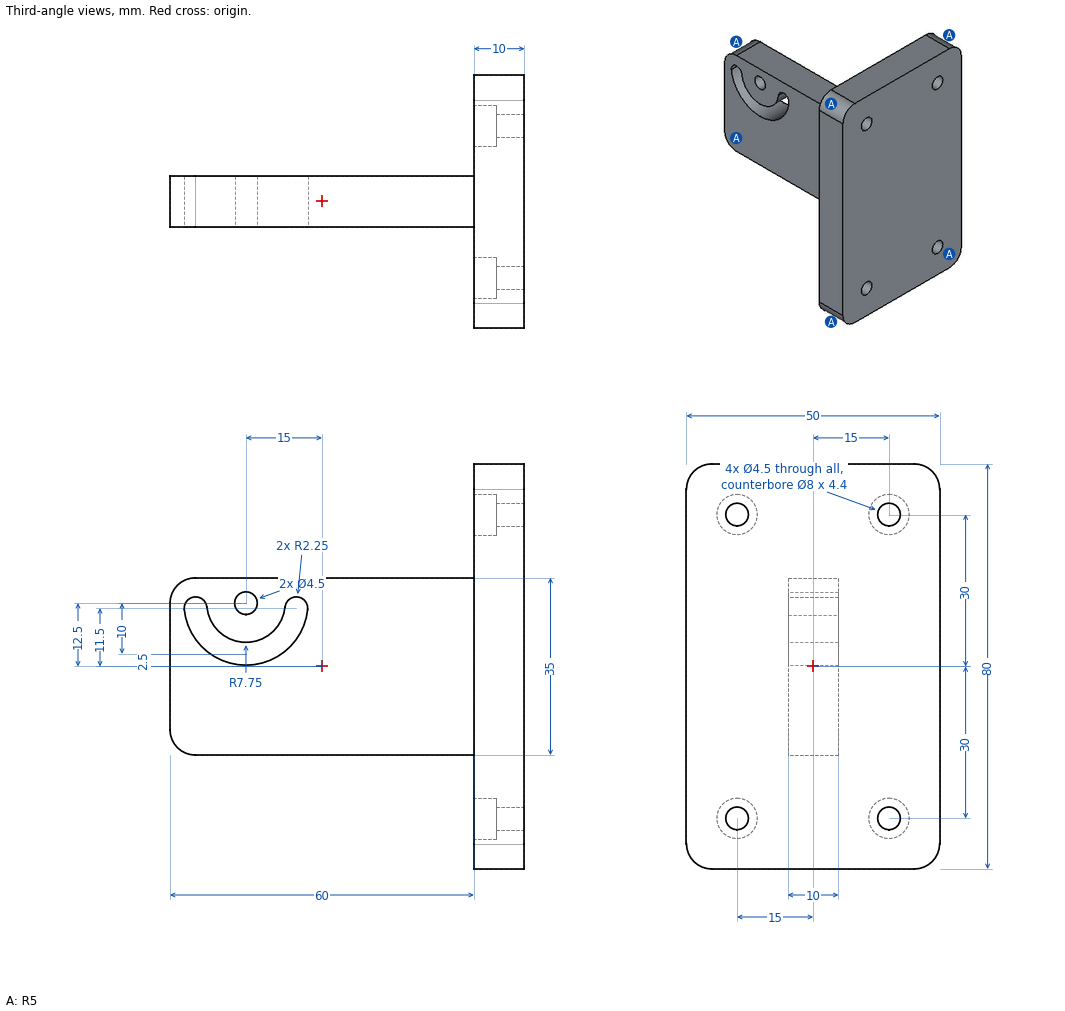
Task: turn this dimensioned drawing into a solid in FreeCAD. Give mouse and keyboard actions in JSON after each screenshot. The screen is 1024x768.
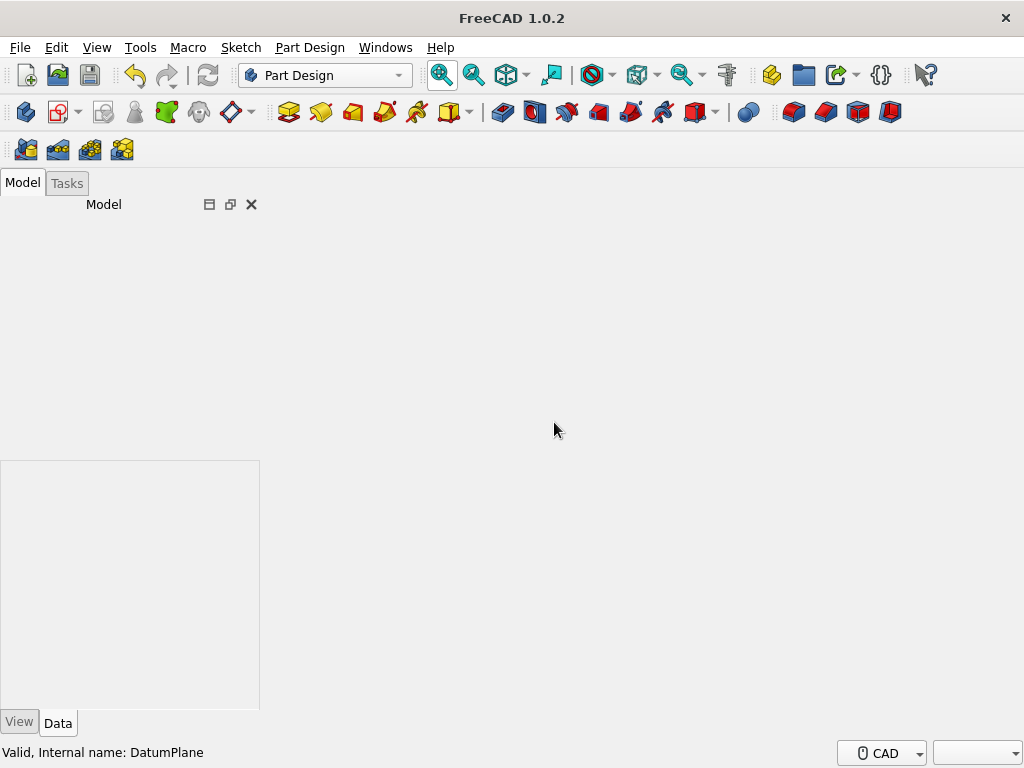
{"action": "left_click", "coordinate": [26, 76]}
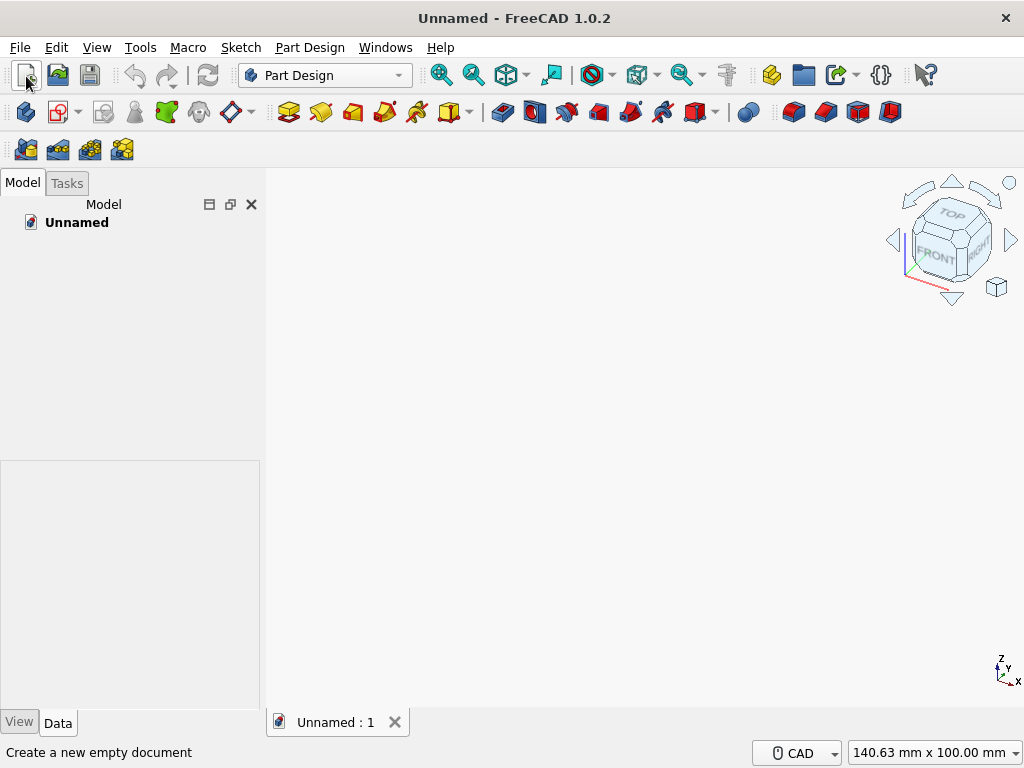
{"action": "left_click", "coordinate": [58, 112]}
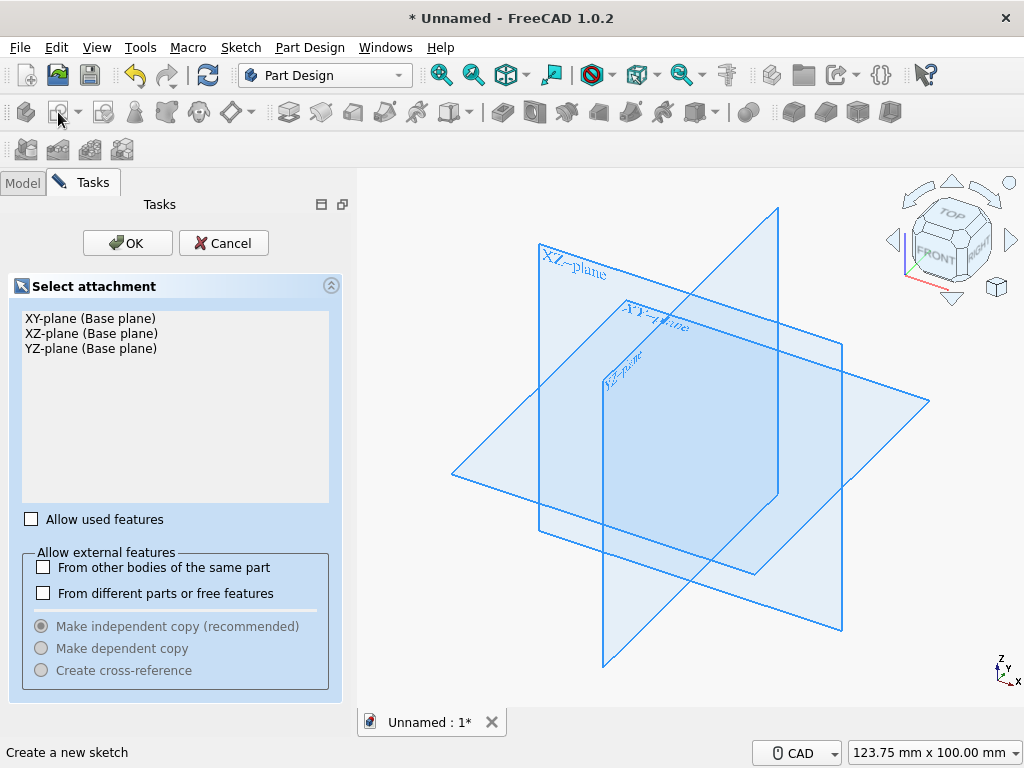
{"action": "left_click", "coordinate": [82, 334]}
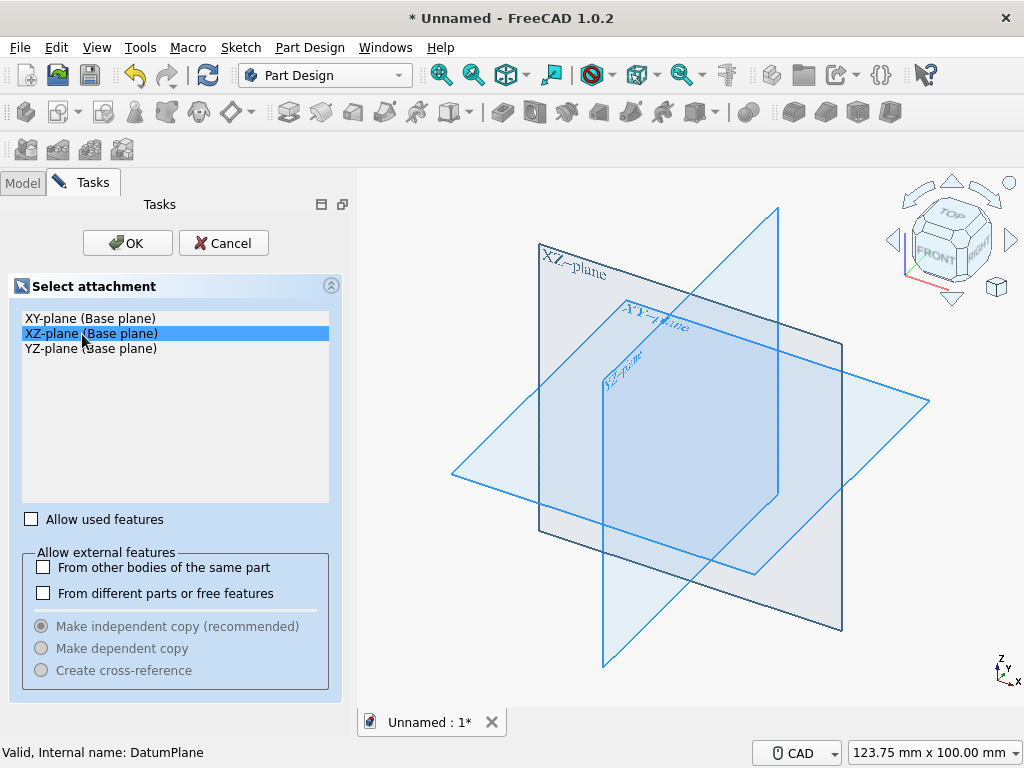
{"action": "left_click", "coordinate": [128, 243]}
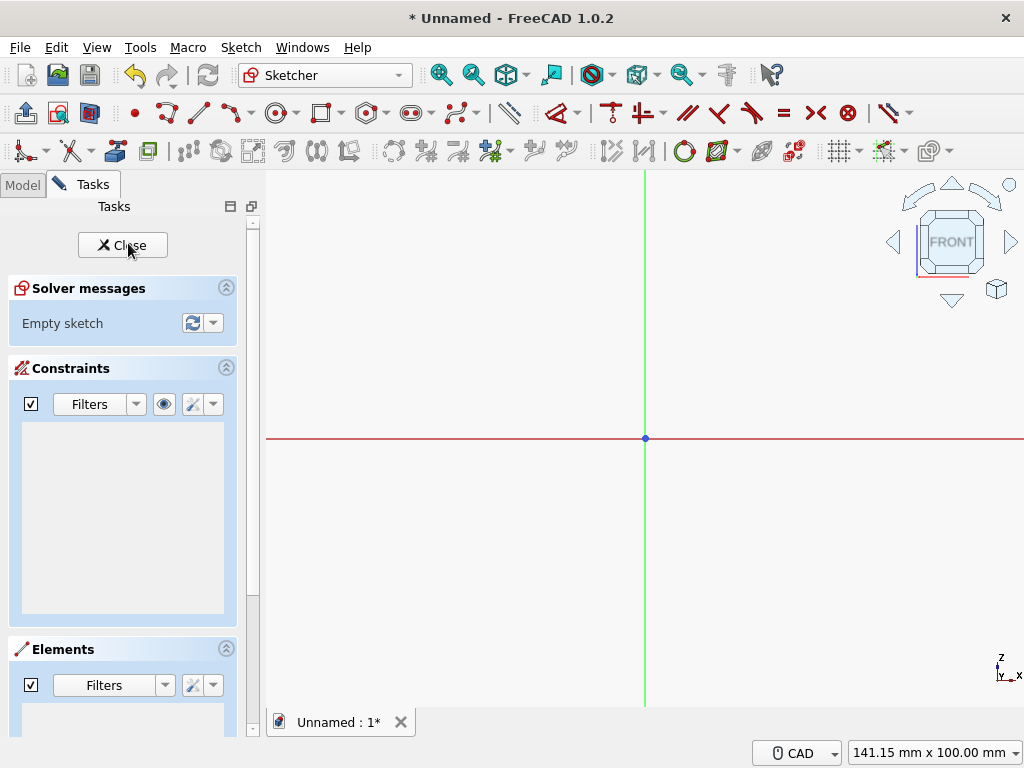
{"action": "left_click", "coordinate": [344, 114]}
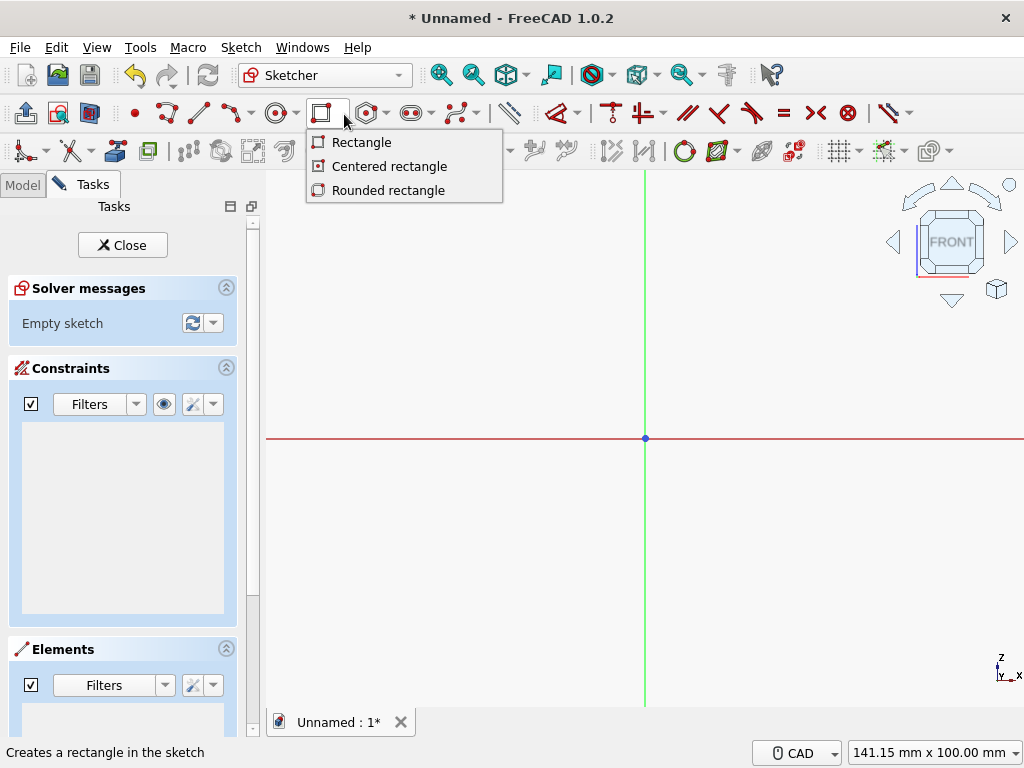
{"action": "left_click", "coordinate": [404, 166]}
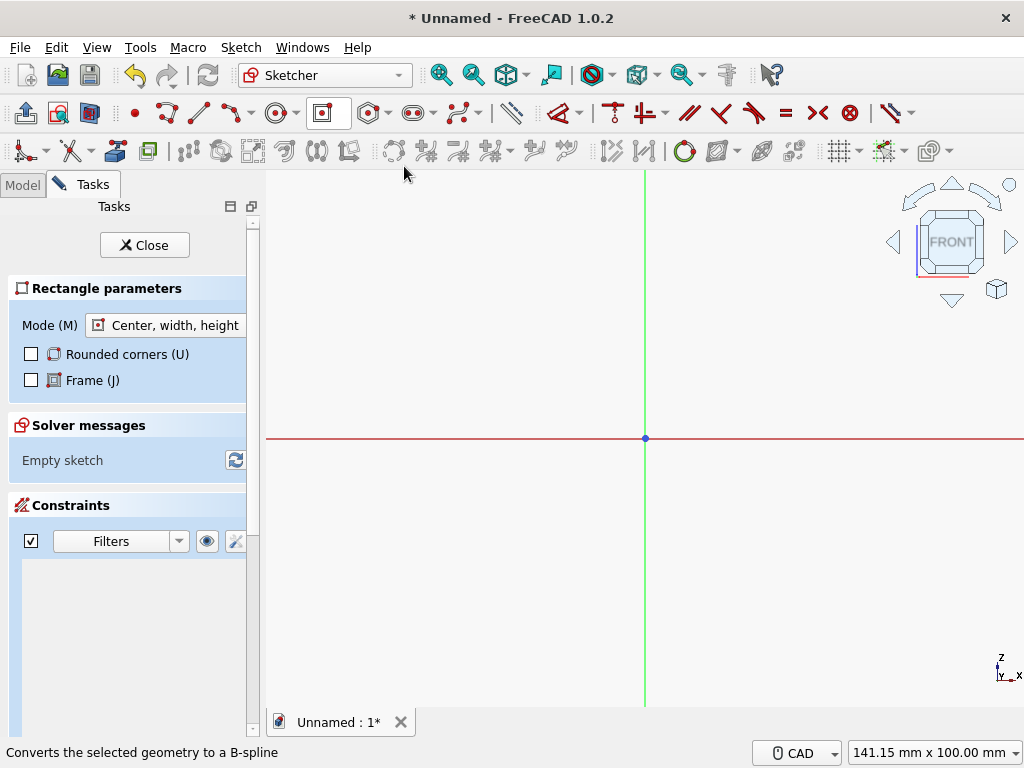
{"action": "left_click", "coordinate": [645, 438]}
{"action": "left_click", "coordinate": [806, 345]}
{"action": "key", "text": "Escape"}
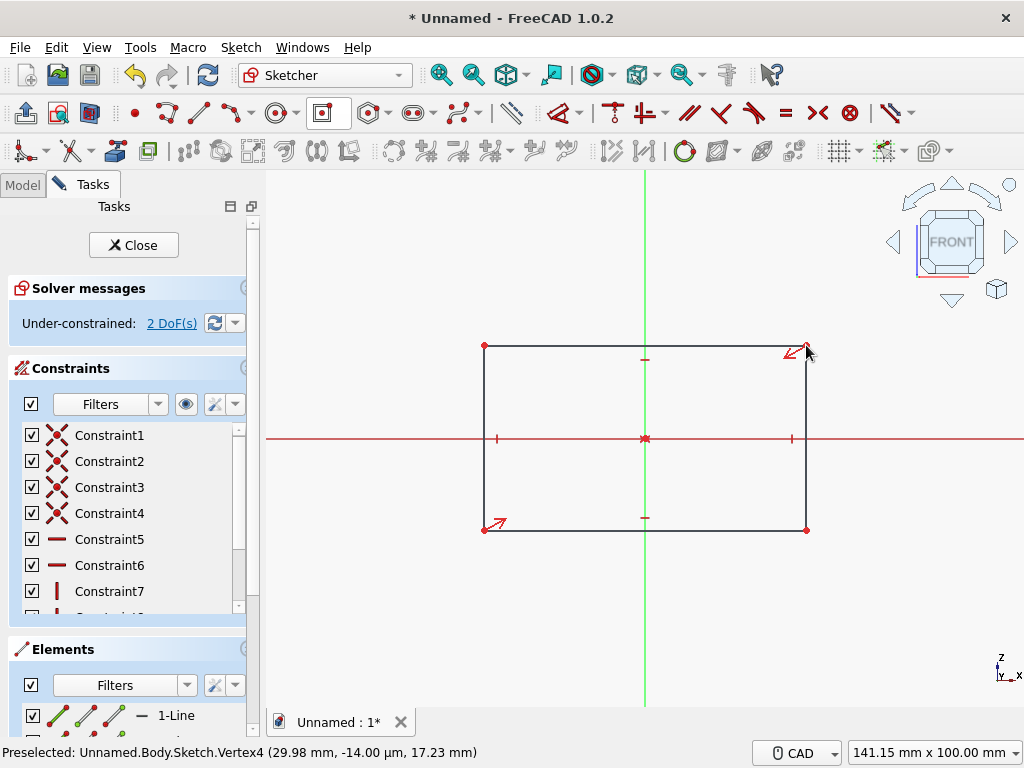
{"action": "left_click", "coordinate": [558, 114]}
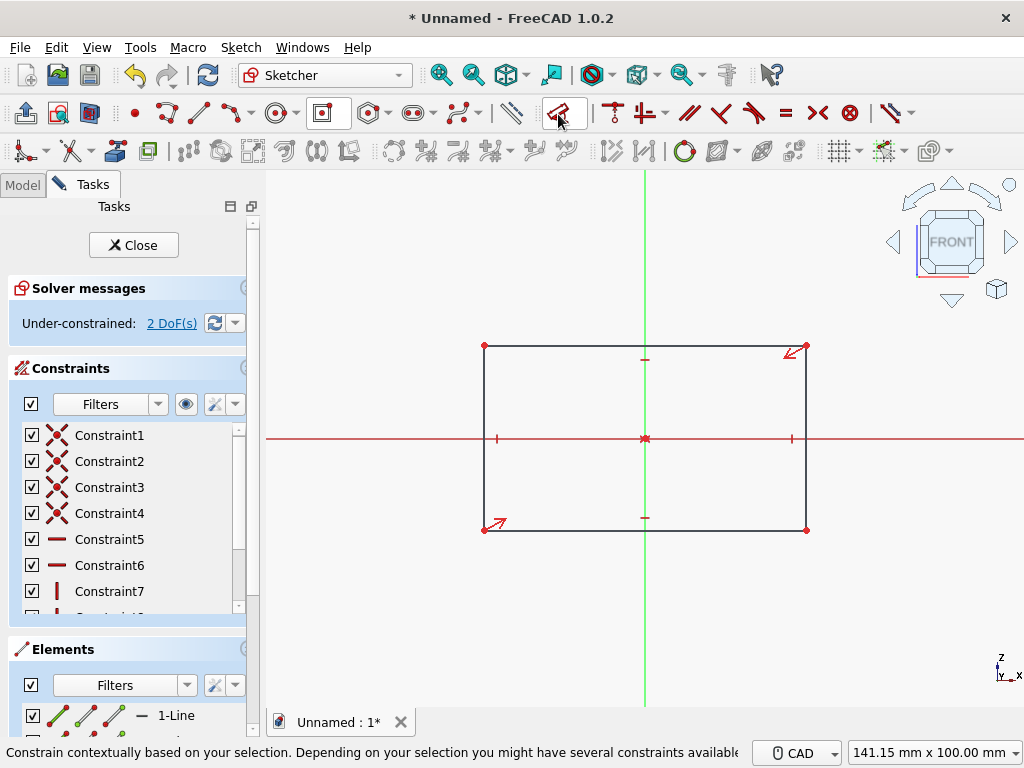
{"action": "left_click", "coordinate": [581, 531]}
{"action": "left_click", "coordinate": [571, 565]}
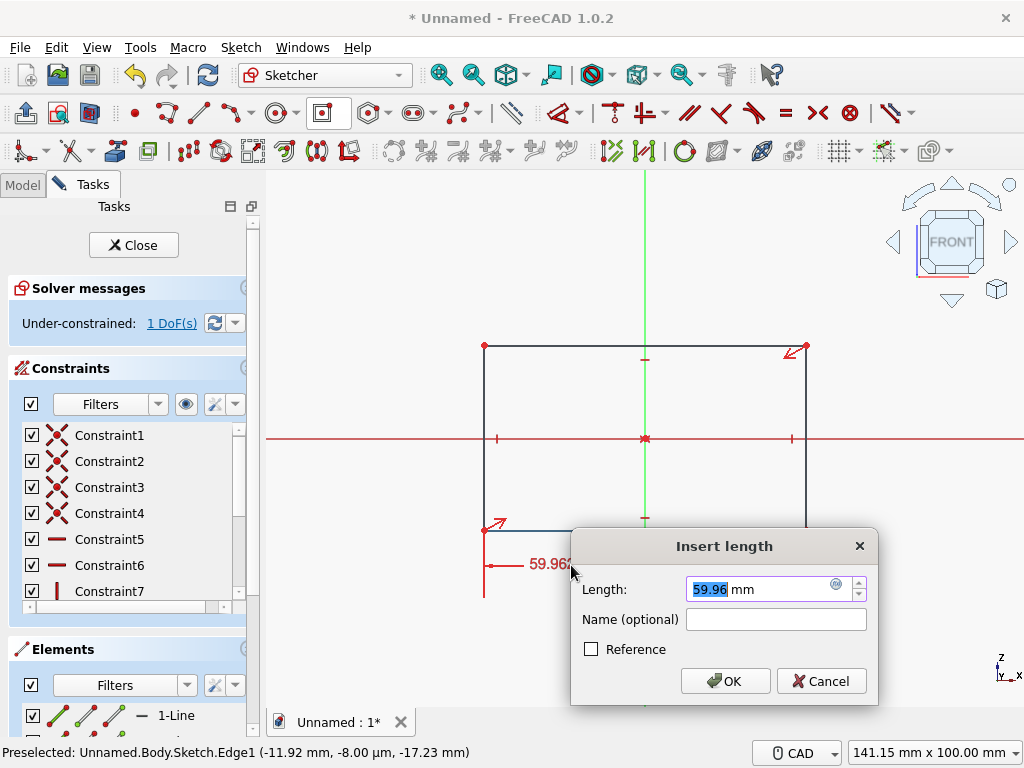
{"action": "type", "text": "60"}
{"action": "key", "text": "Return"}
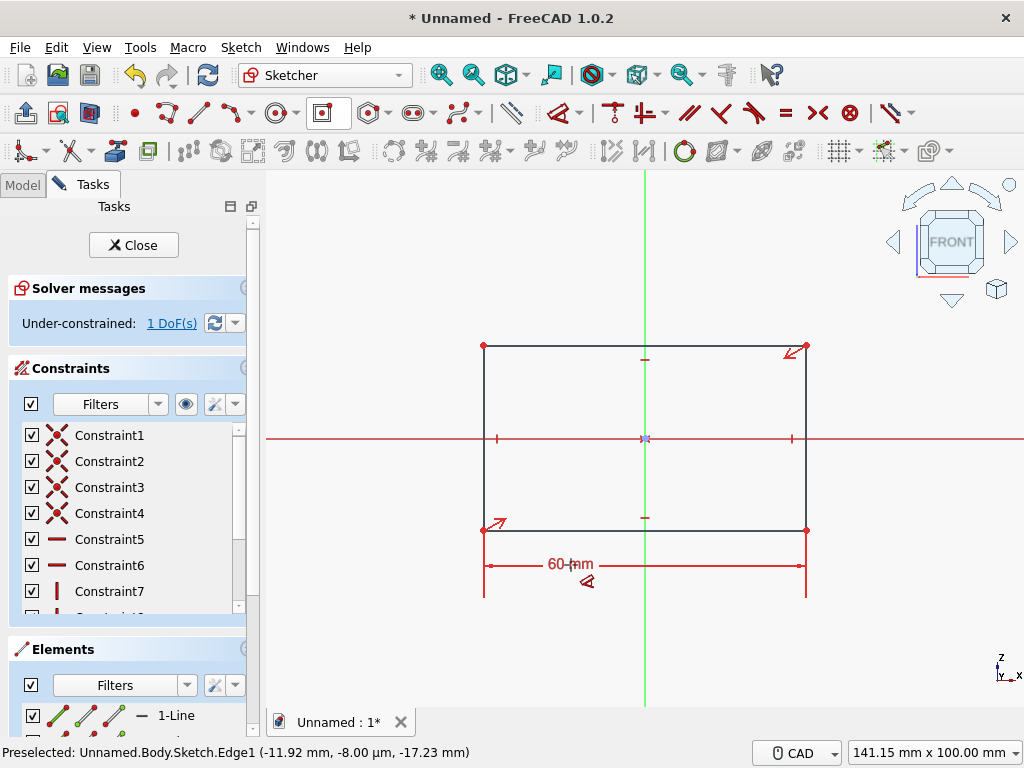
{"action": "left_click", "coordinate": [806, 475]}
{"action": "left_click", "coordinate": [840, 396]}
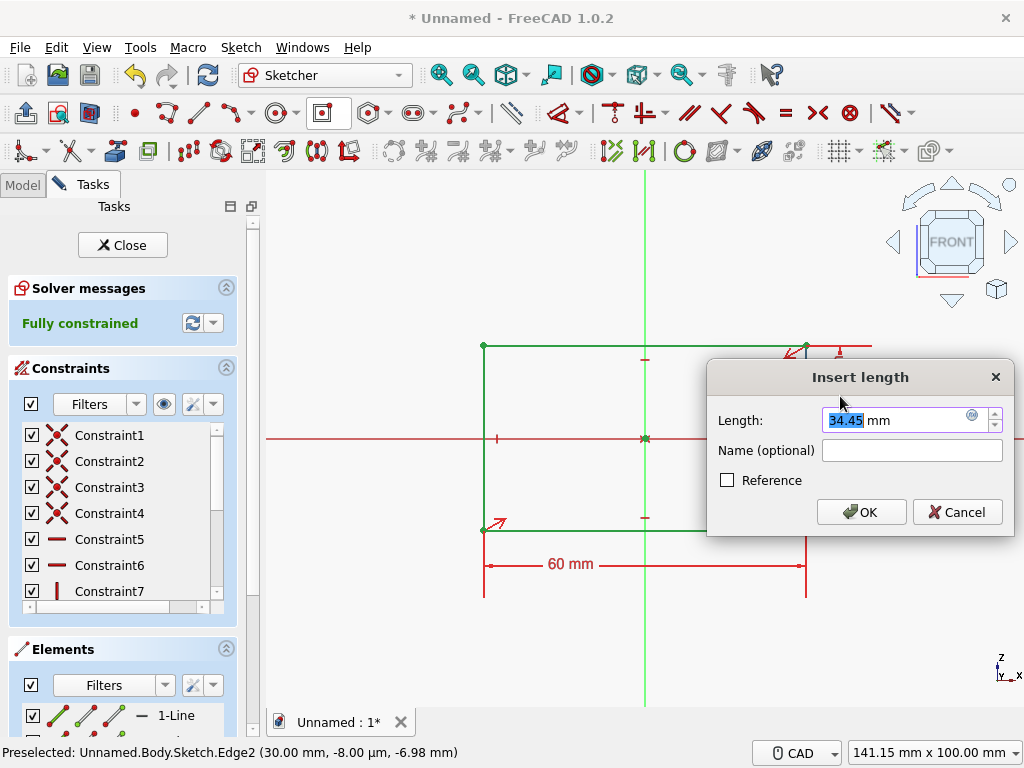
{"action": "type", "text": "35"}
{"action": "key", "text": "Return"}
{"action": "key", "text": "Escape"}